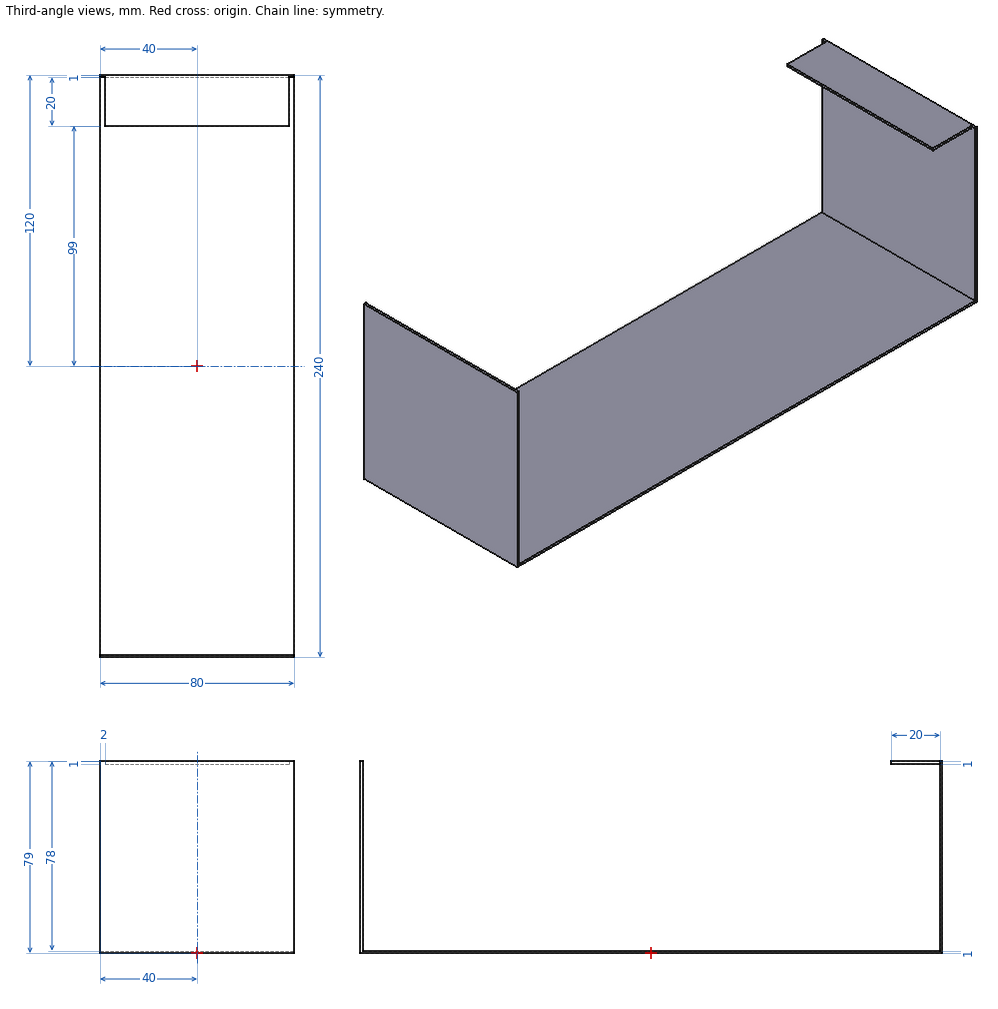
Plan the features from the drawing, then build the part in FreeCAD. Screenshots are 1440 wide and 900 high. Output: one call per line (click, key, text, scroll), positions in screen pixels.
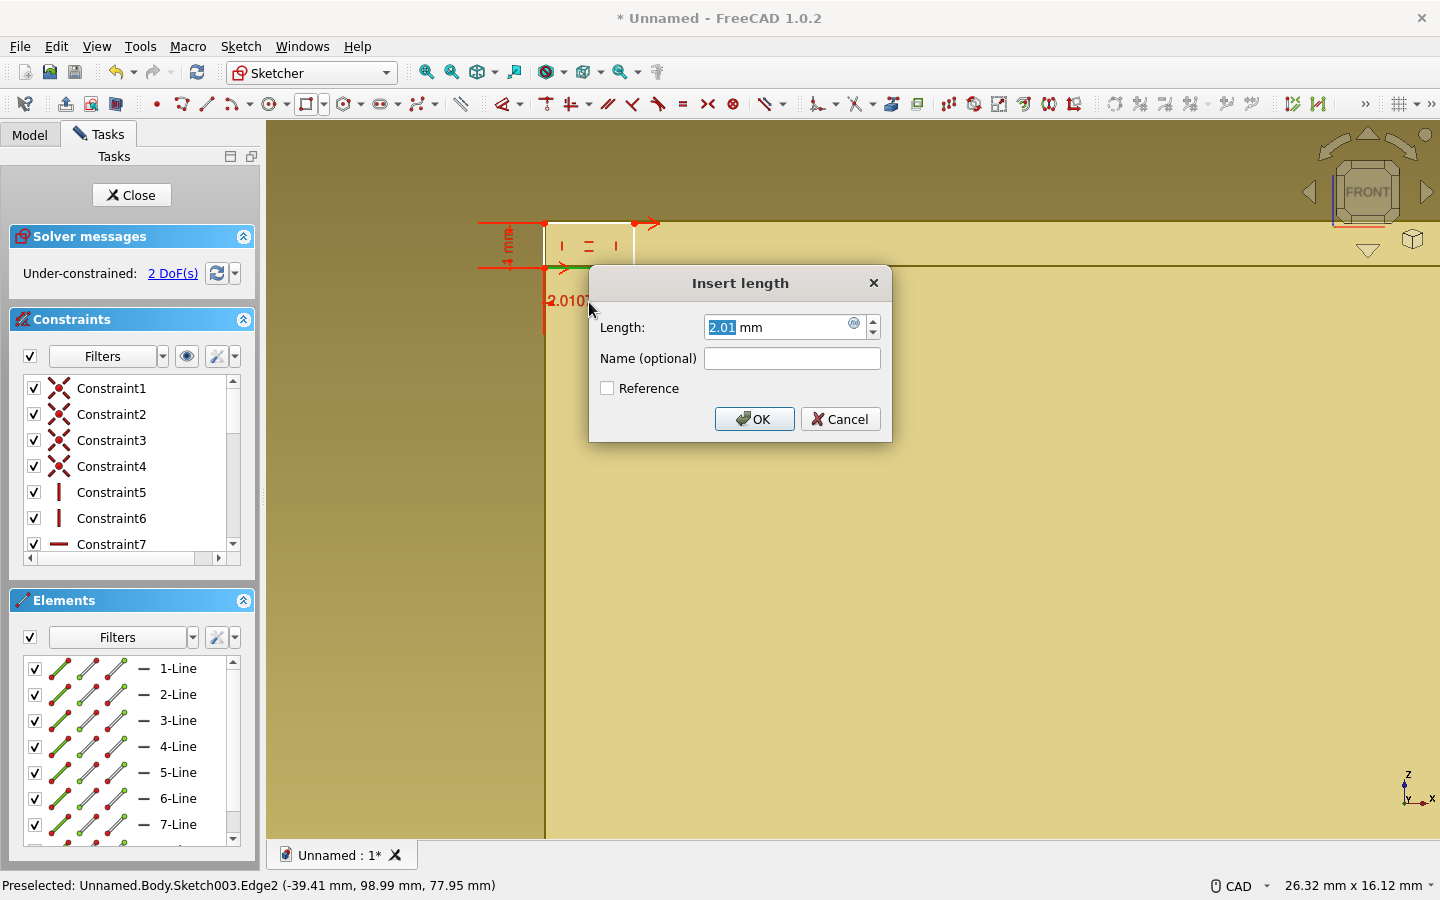
text(2)
key(Return)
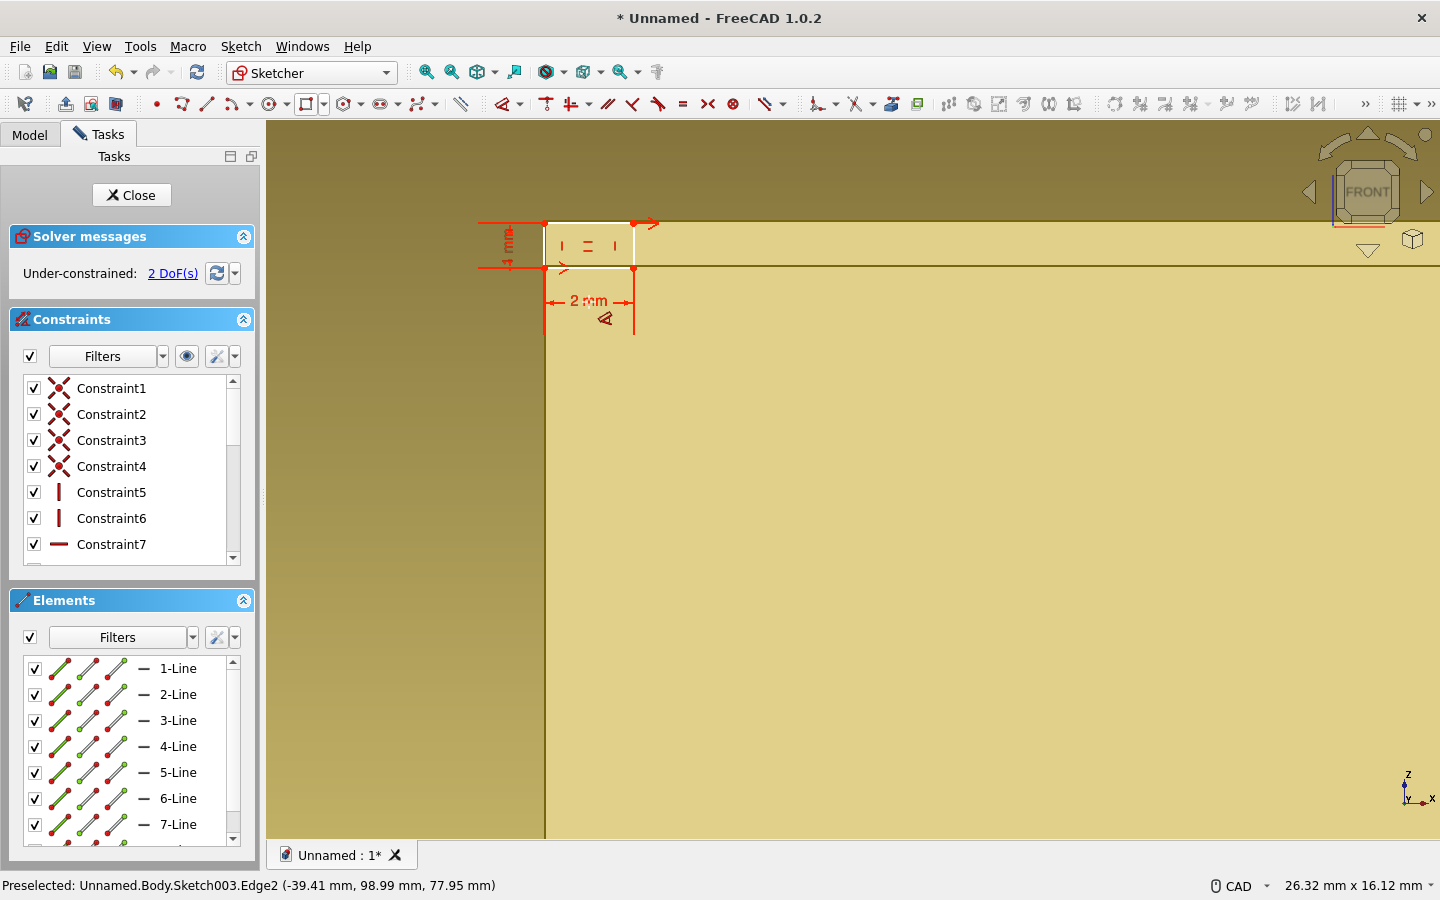
scroll(543, 244, down, 10)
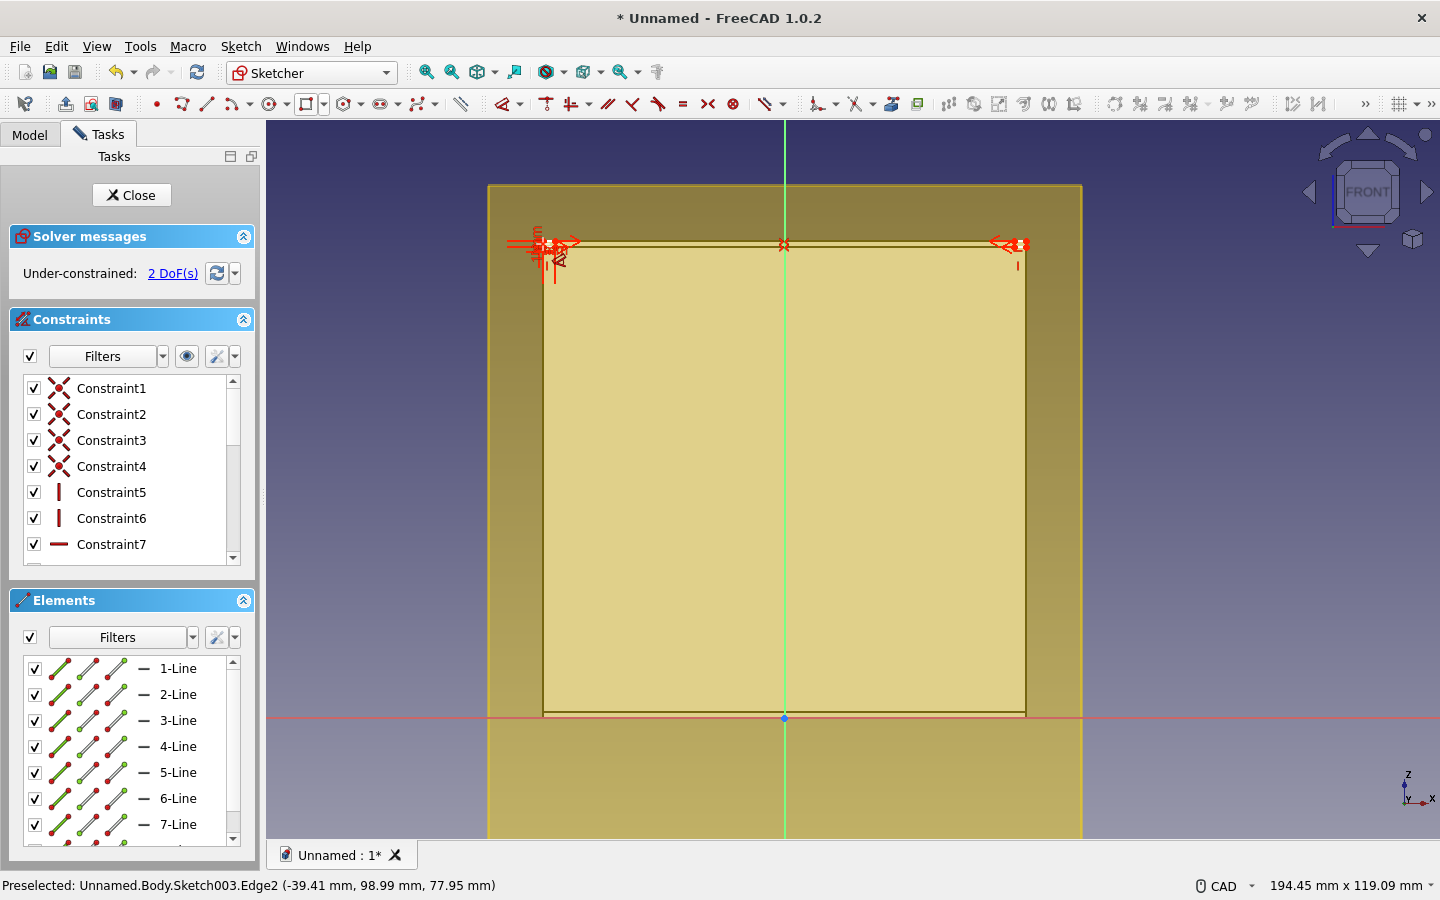
scroll(543, 241, up, 4)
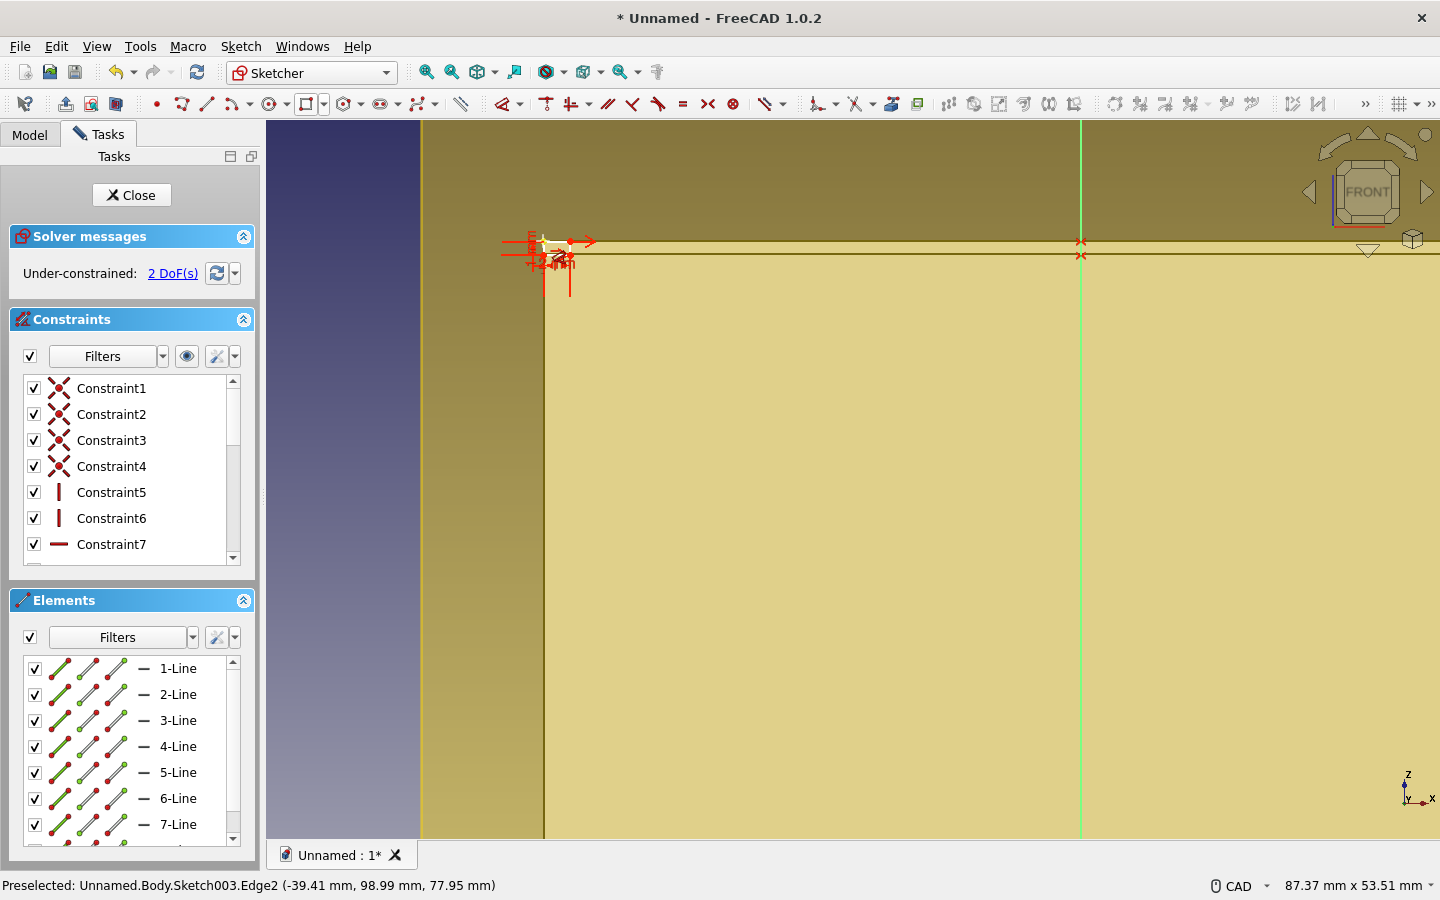
click(544, 242)
click(812, 208)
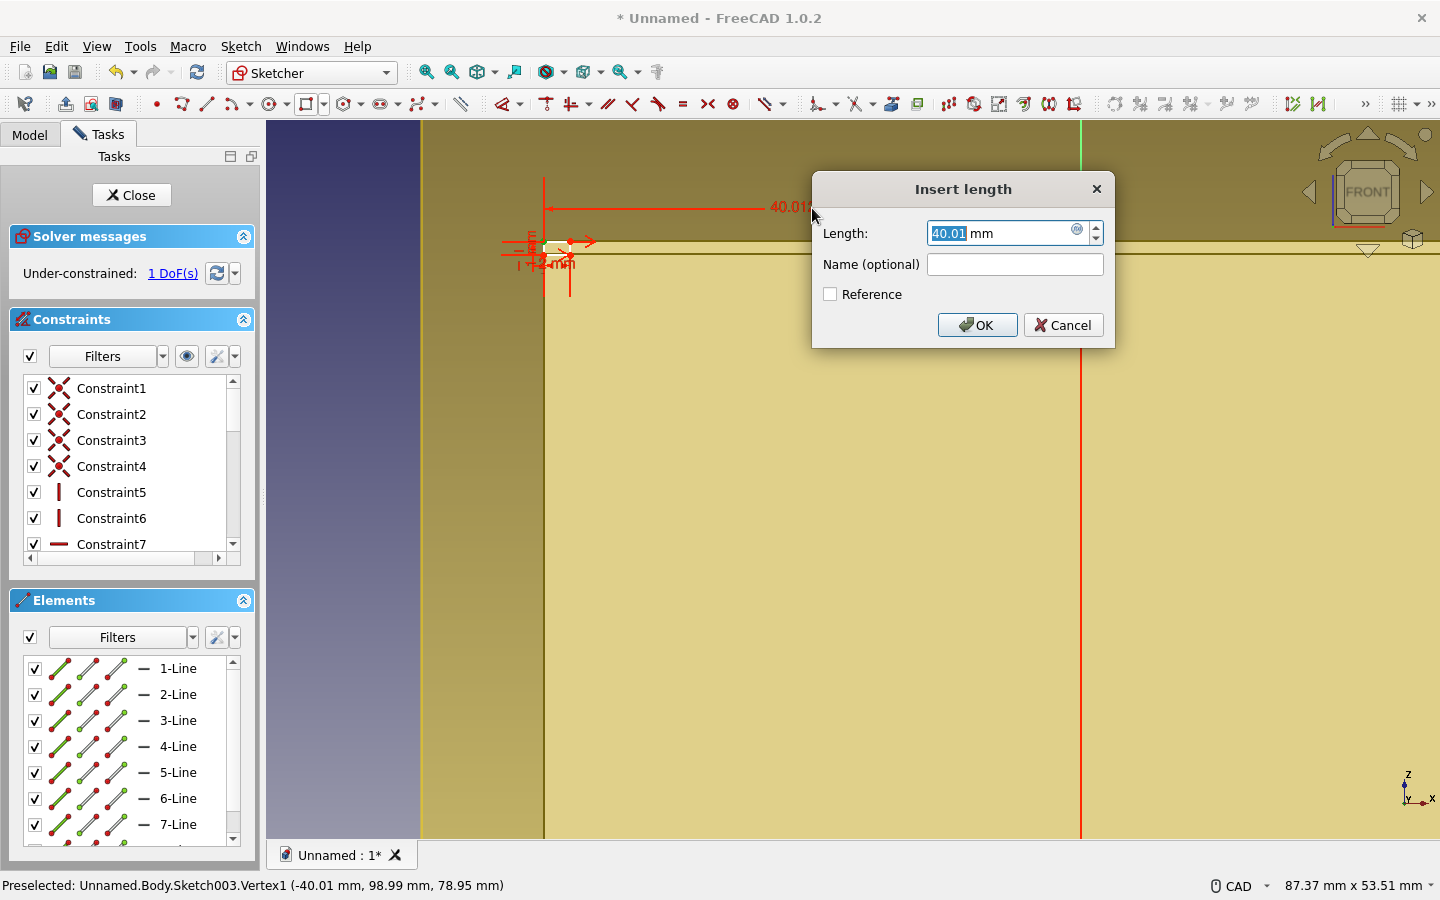
text(40)
key(Return)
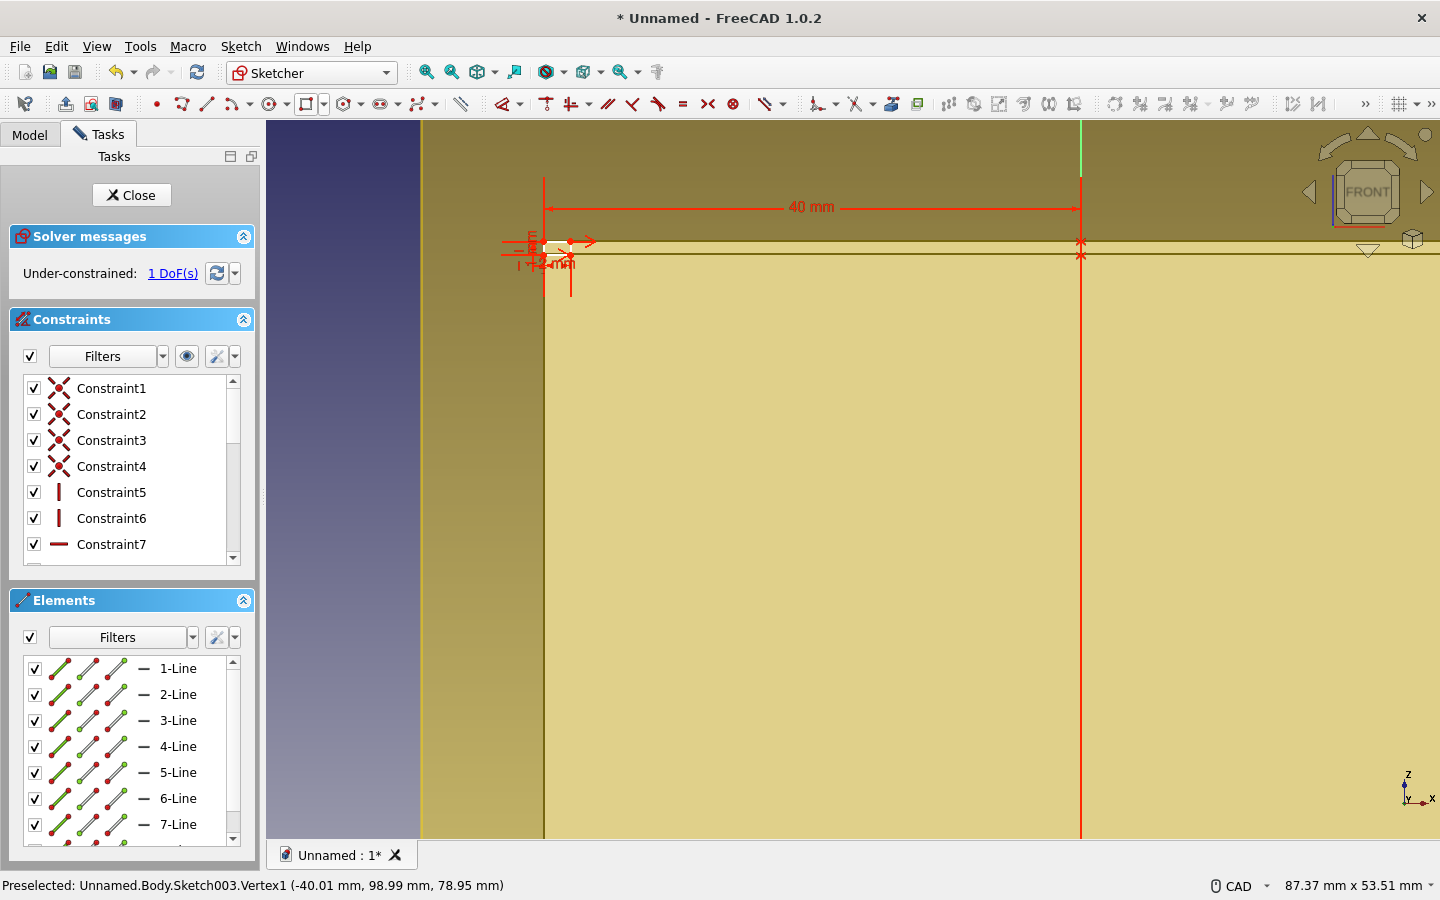
click(544, 242)
click(510, 526)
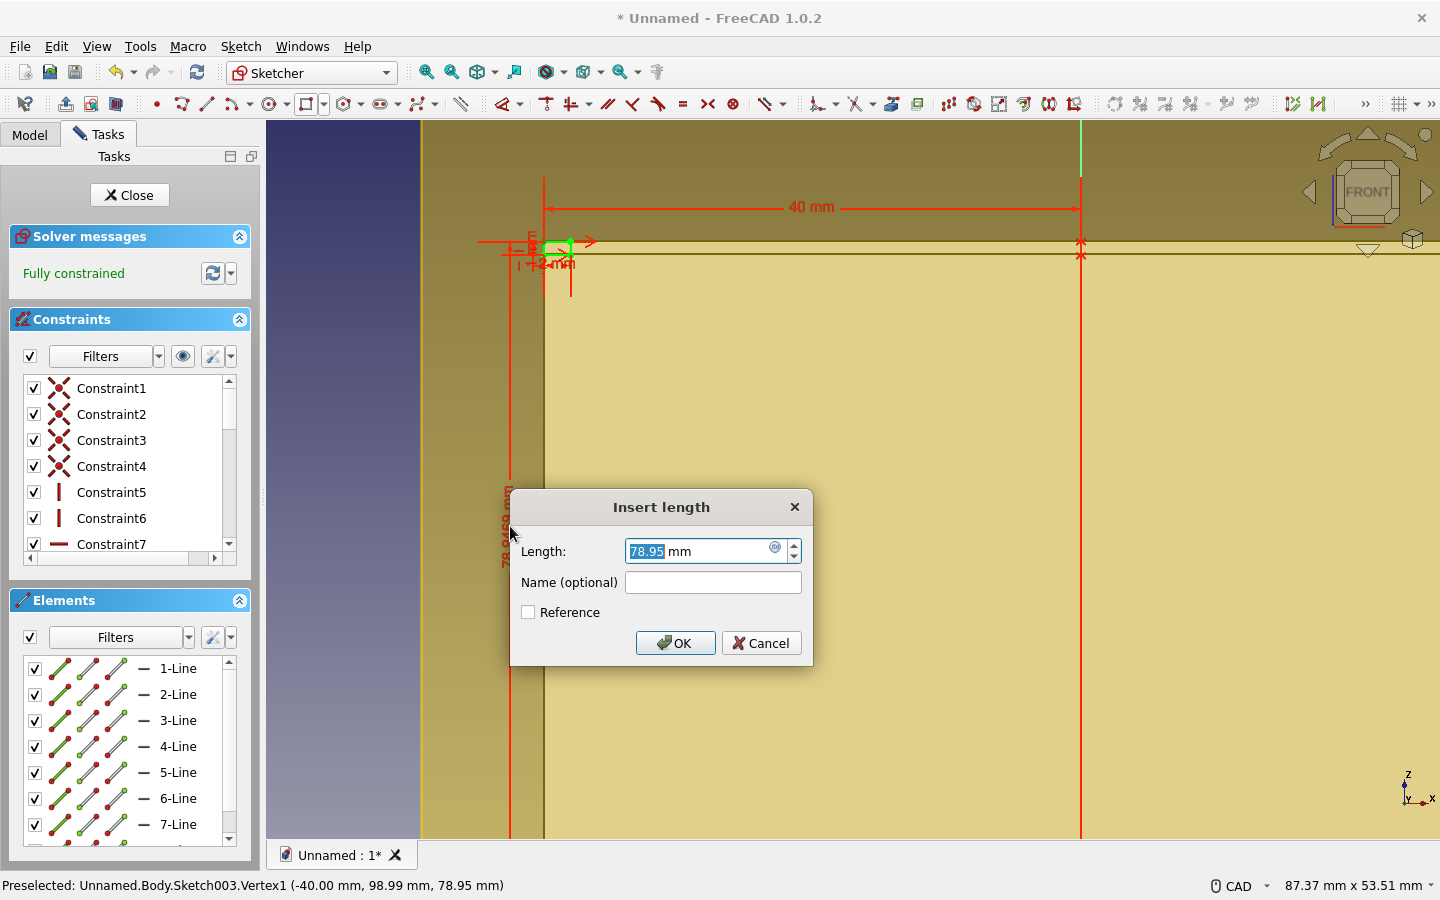
text(79)
key(Return)
key(Escape)